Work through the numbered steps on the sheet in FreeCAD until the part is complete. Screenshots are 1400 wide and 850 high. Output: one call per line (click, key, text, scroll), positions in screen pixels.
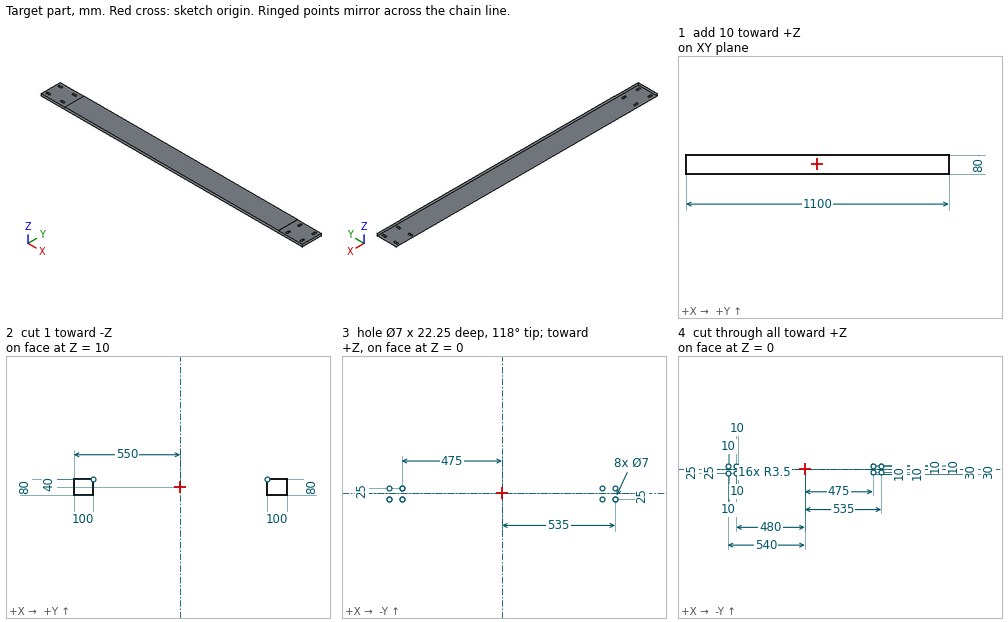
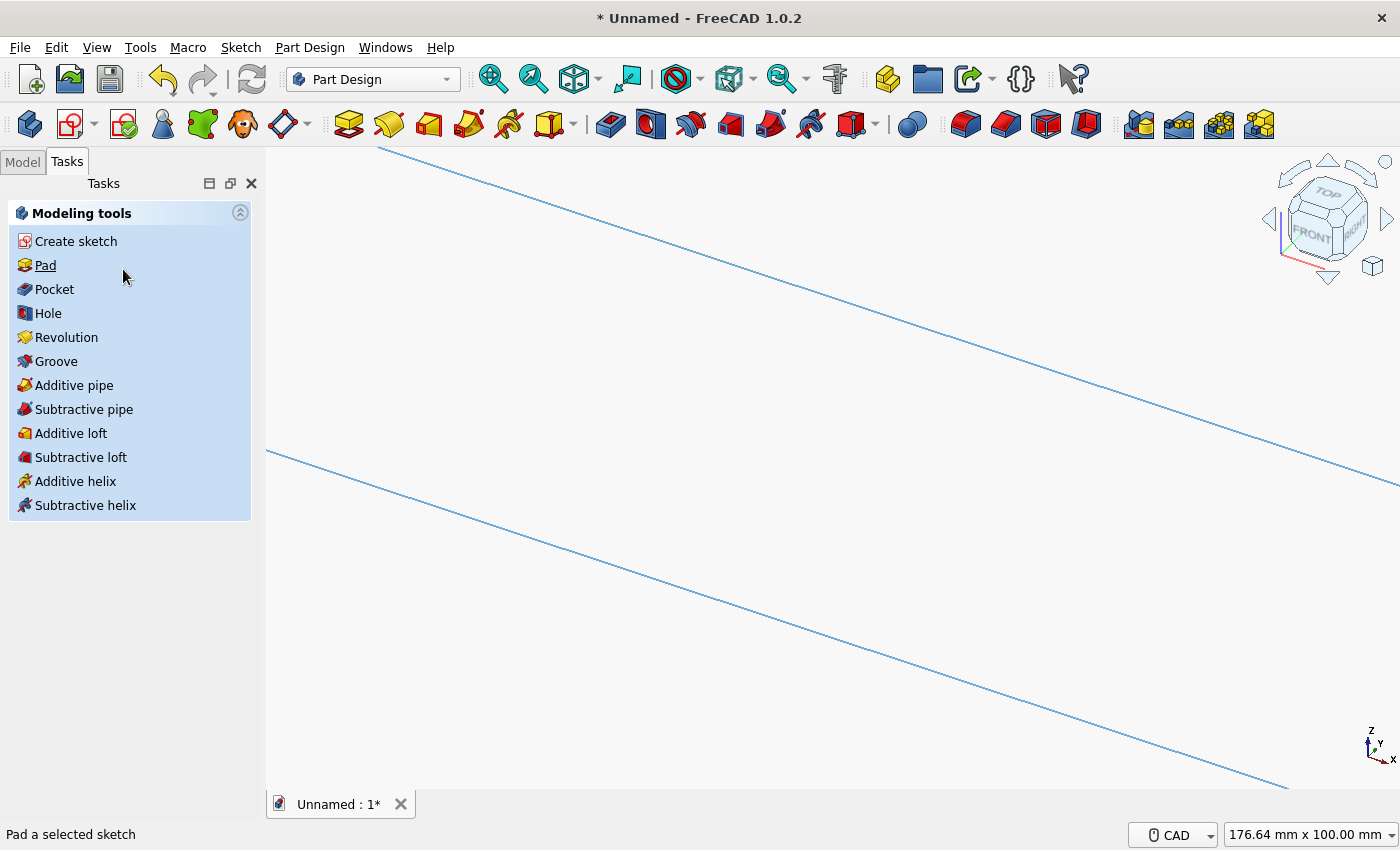
click(350, 124)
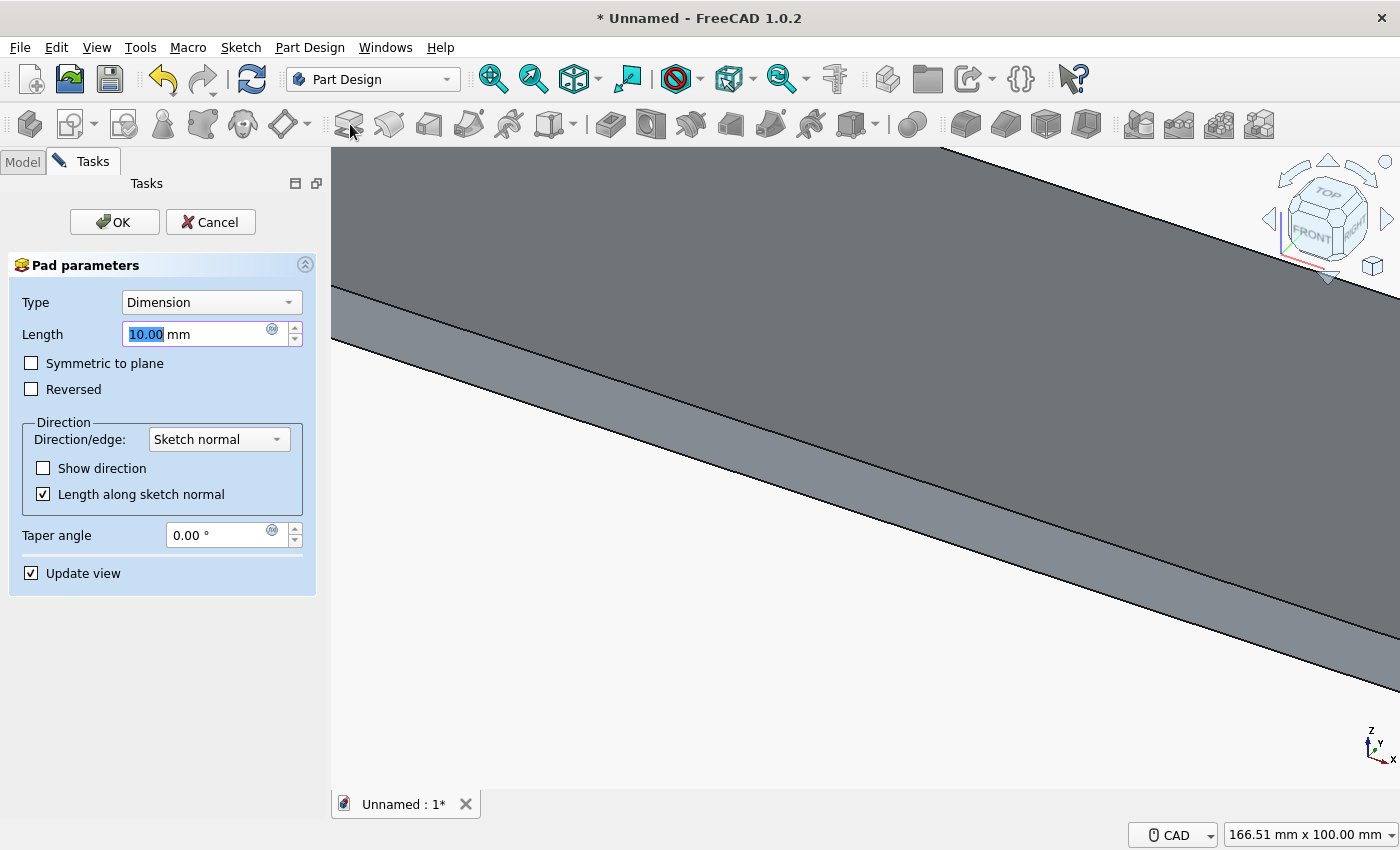
text(10)
key(Tab)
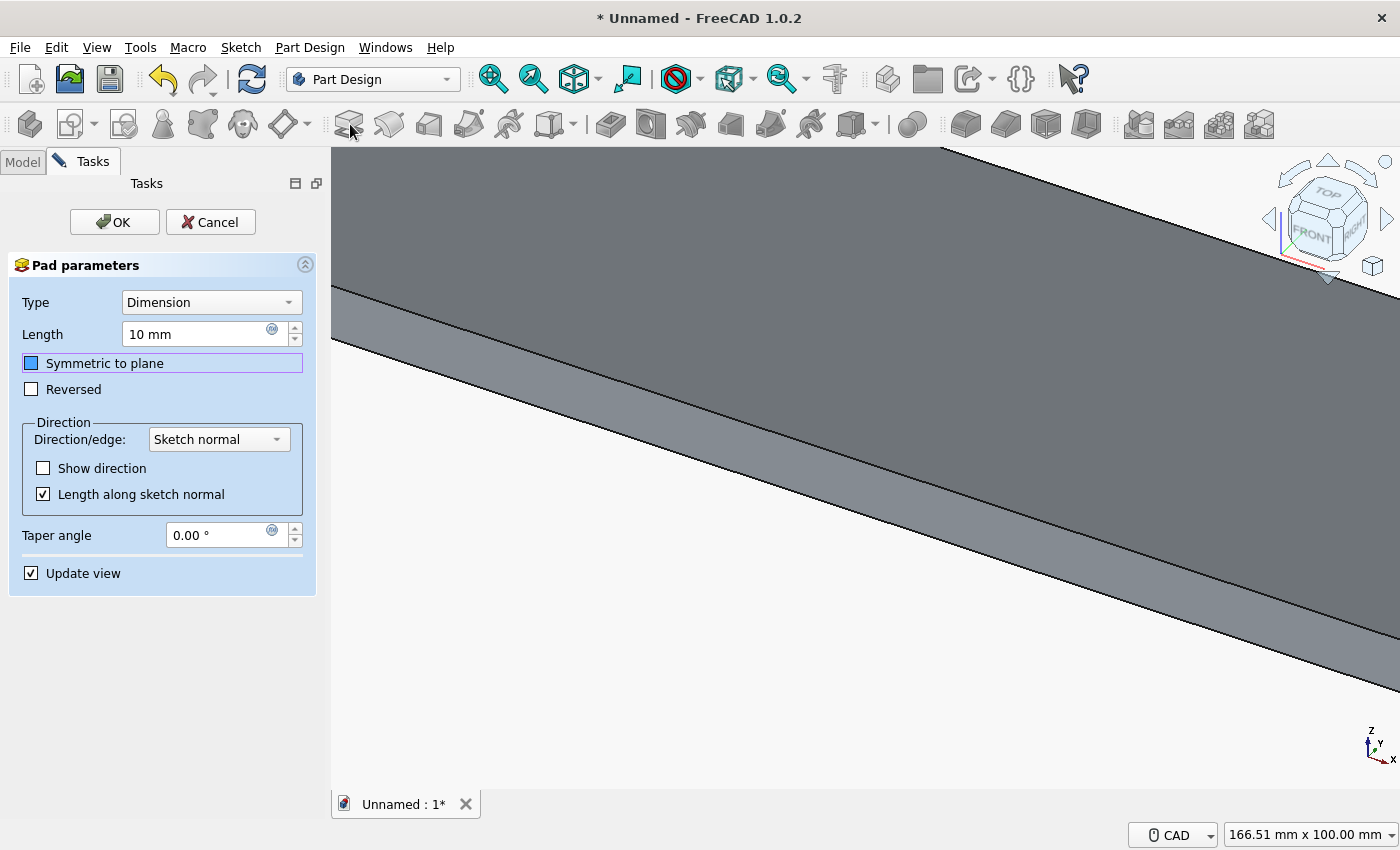
click(115, 222)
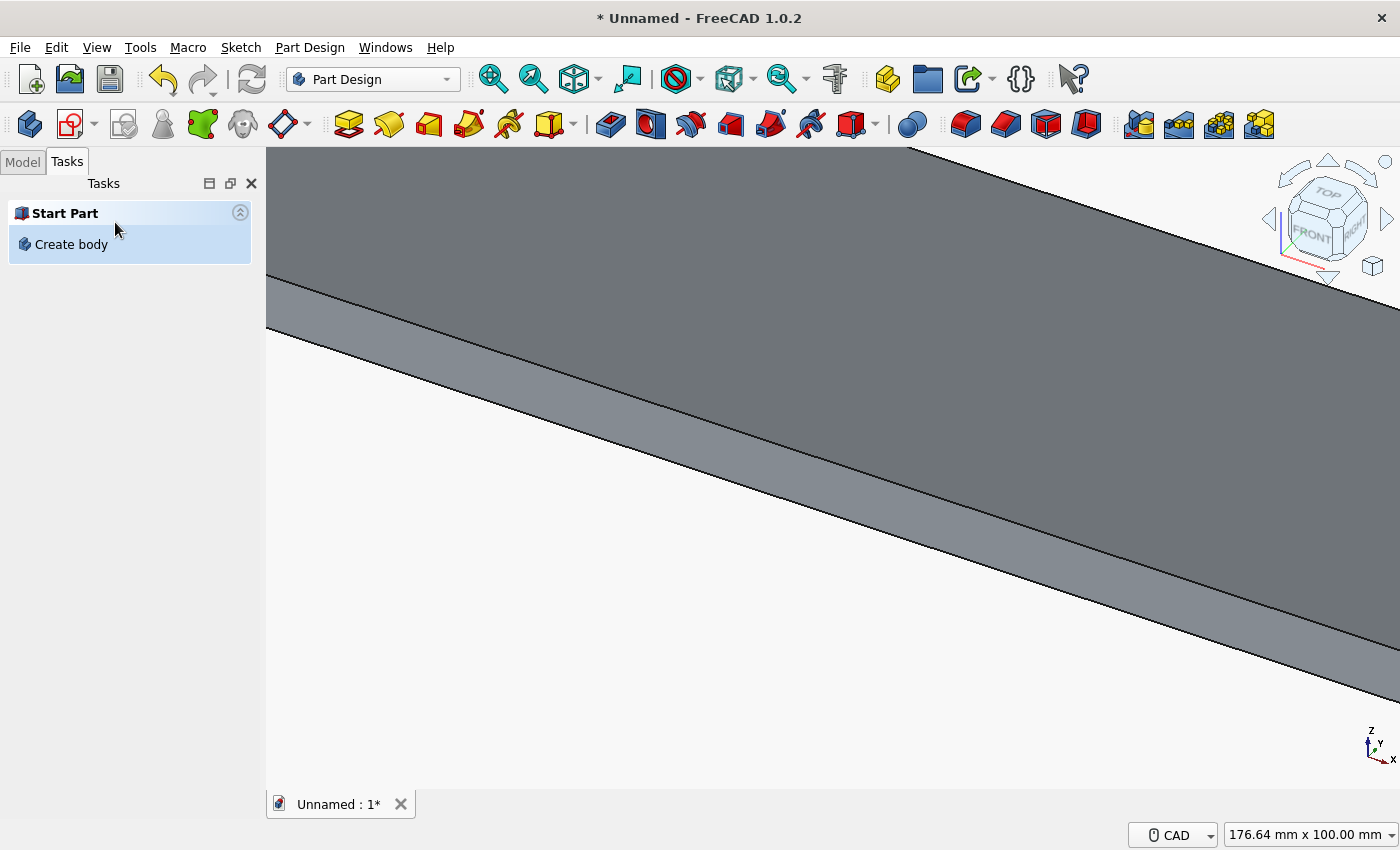
click(494, 80)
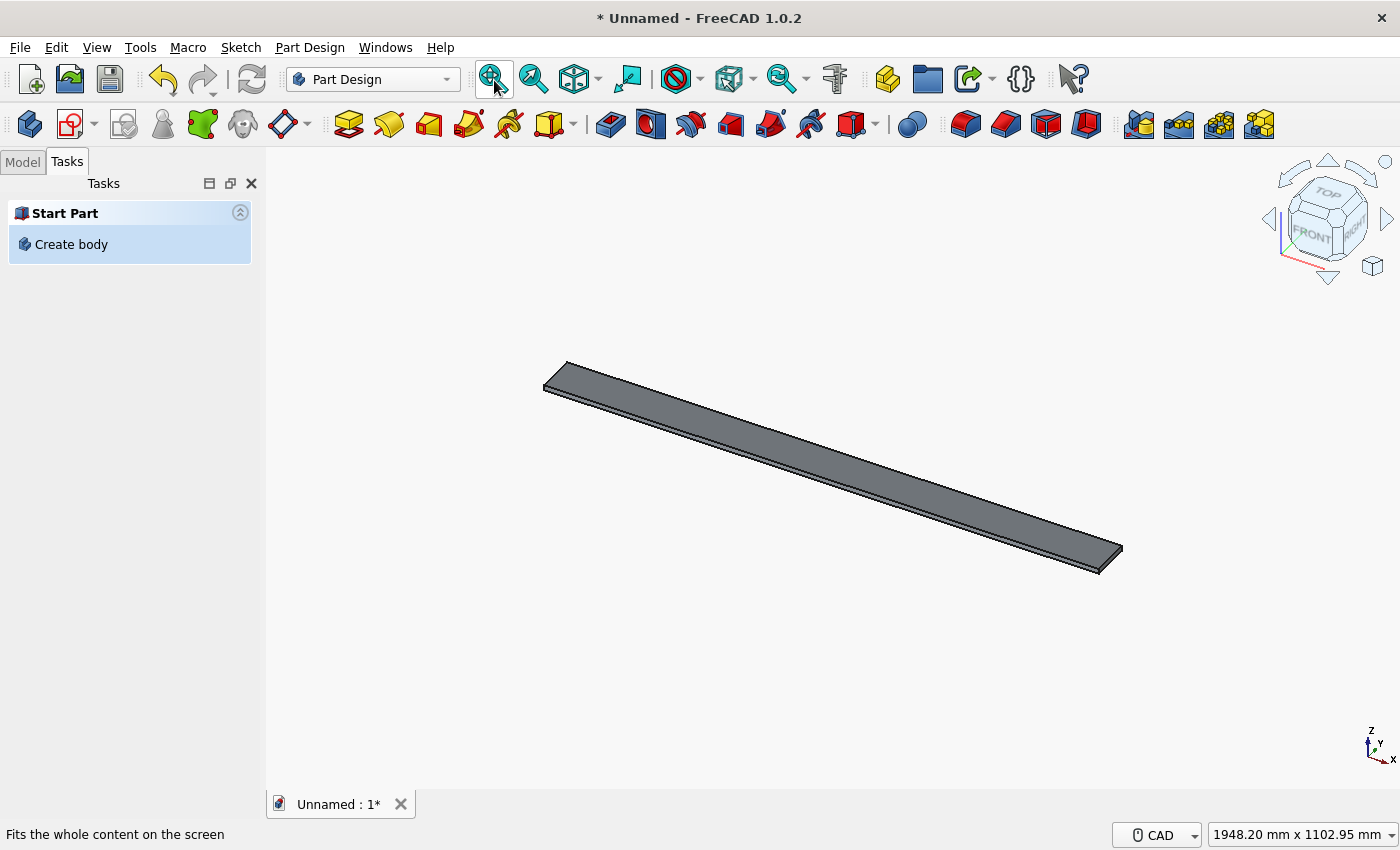
click(1071, 543)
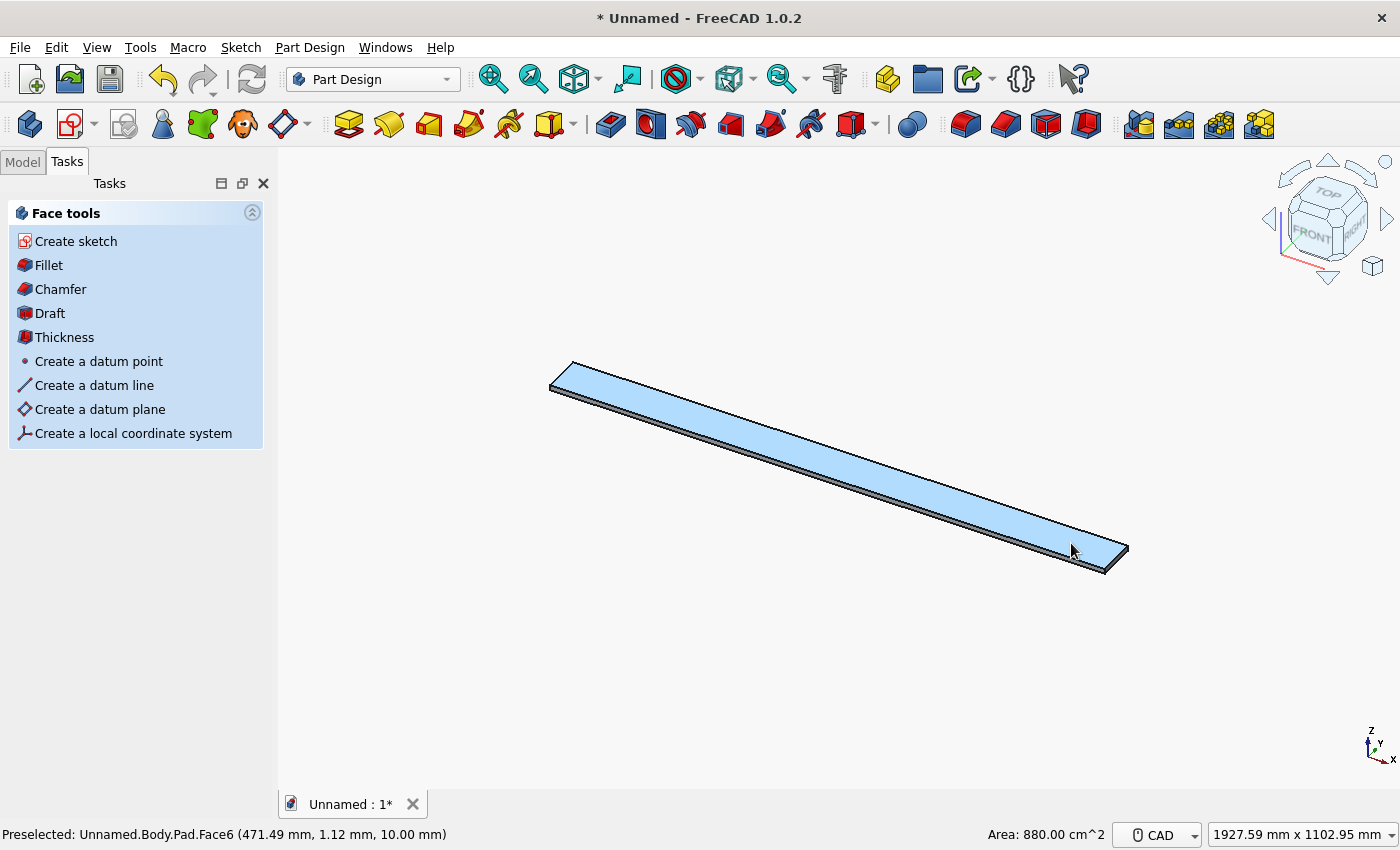
click(70, 124)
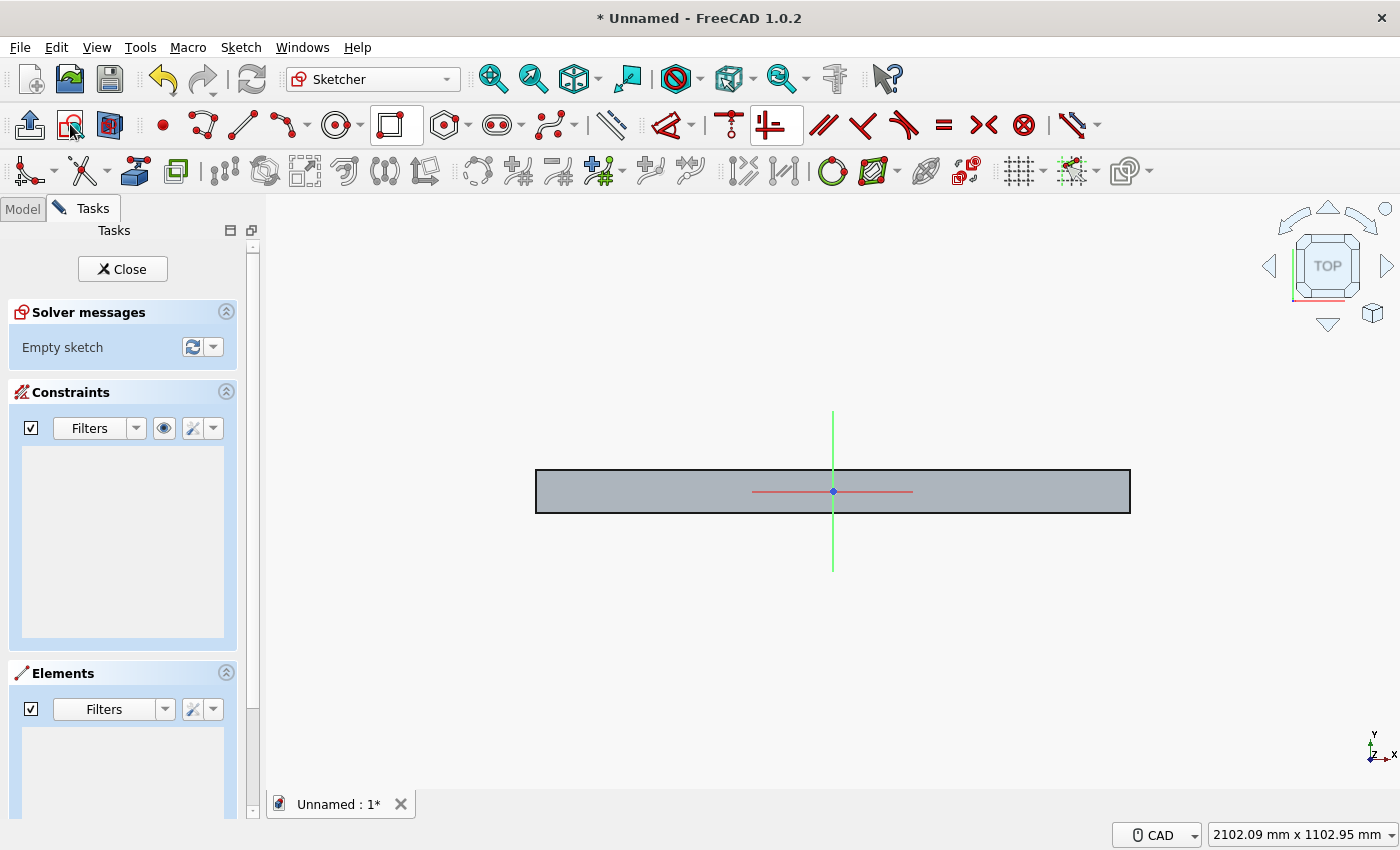
click(390, 126)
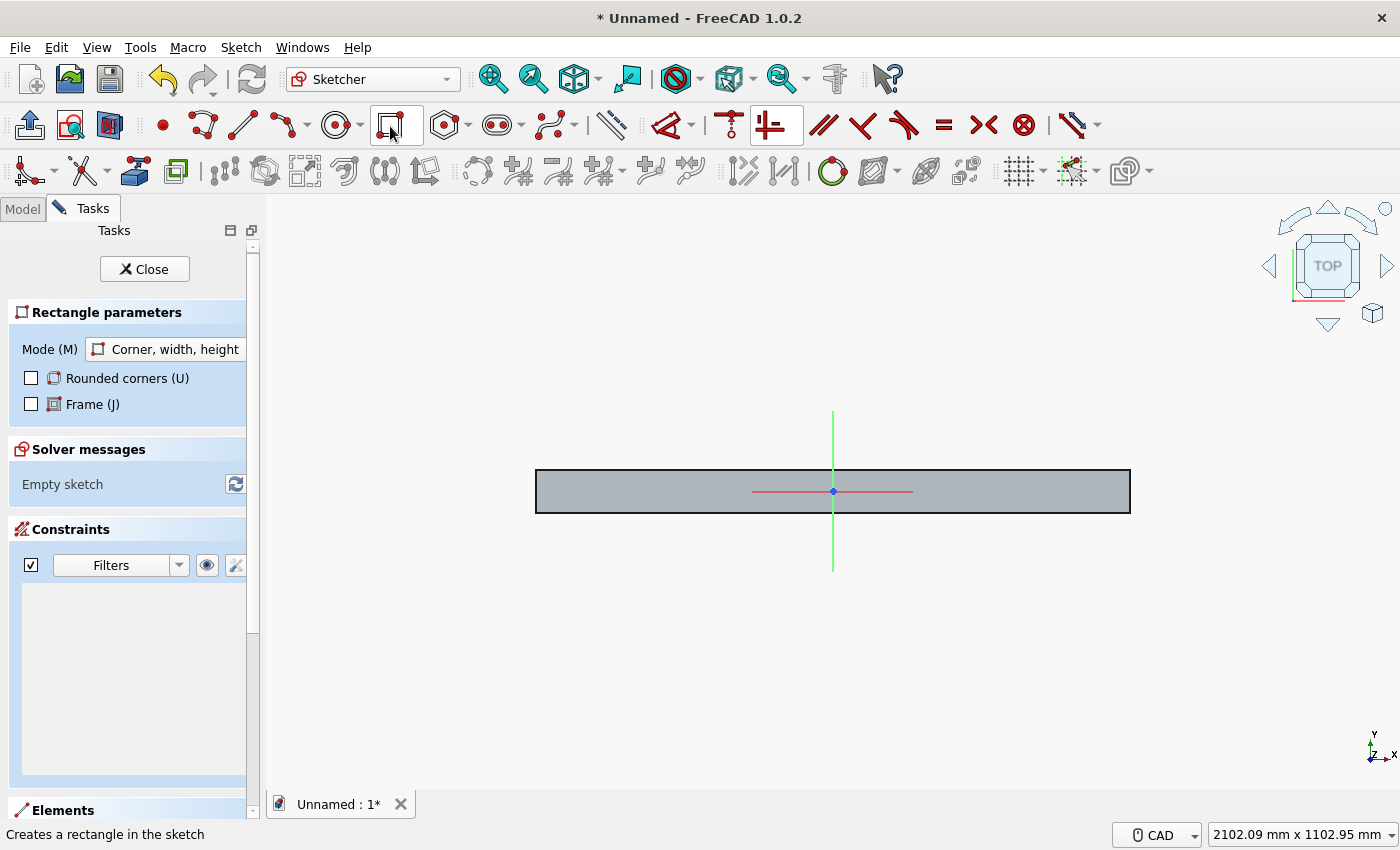
click(536, 470)
move(590, 513)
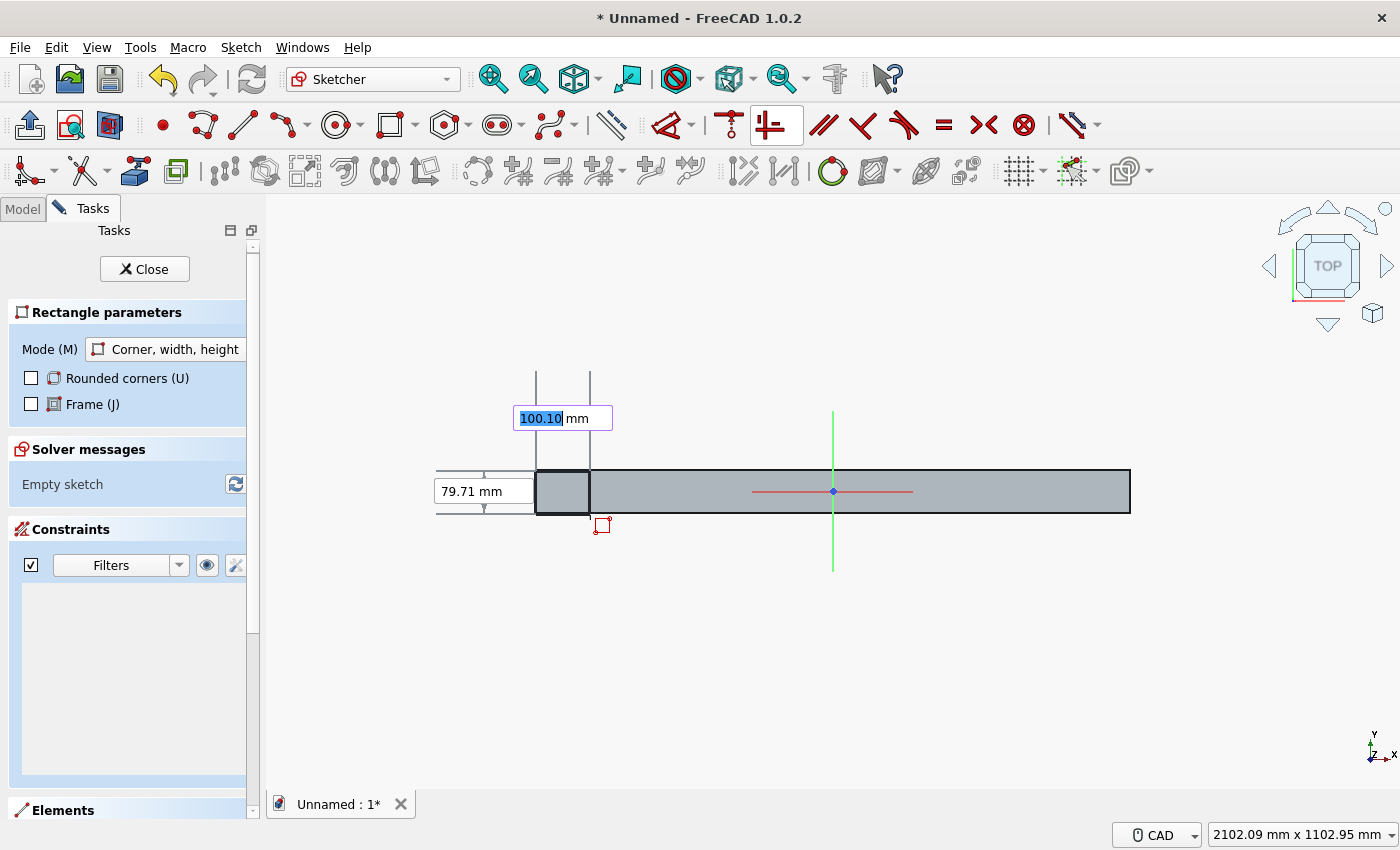
text(100)
key(Tab)
text(80)
key(Return)